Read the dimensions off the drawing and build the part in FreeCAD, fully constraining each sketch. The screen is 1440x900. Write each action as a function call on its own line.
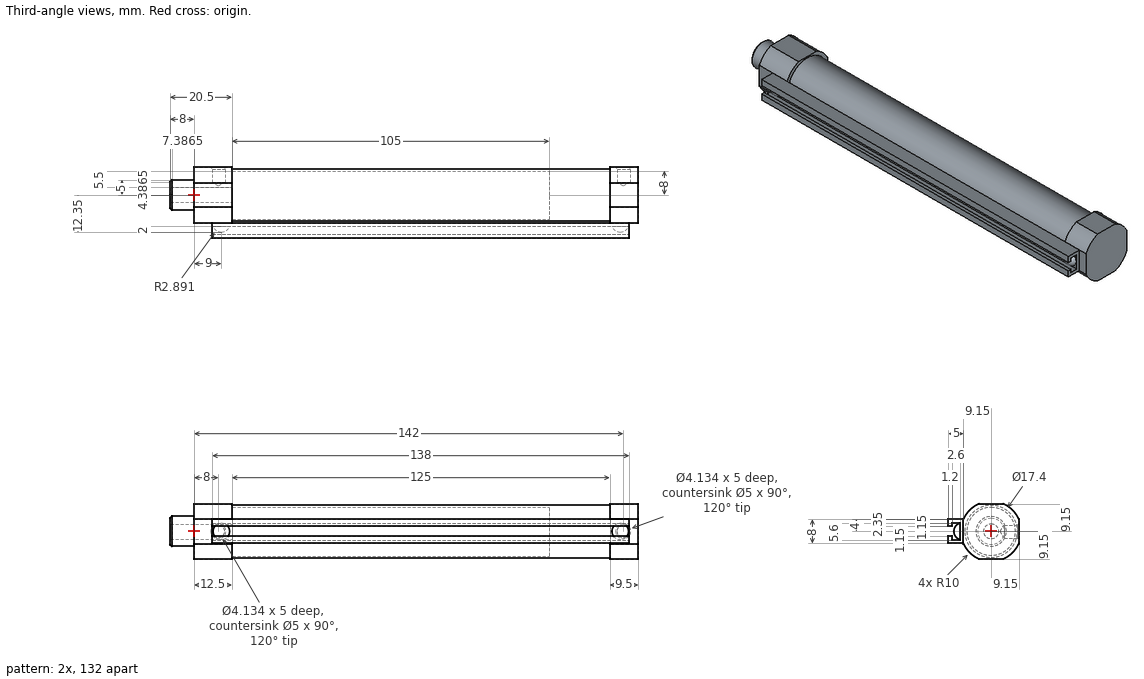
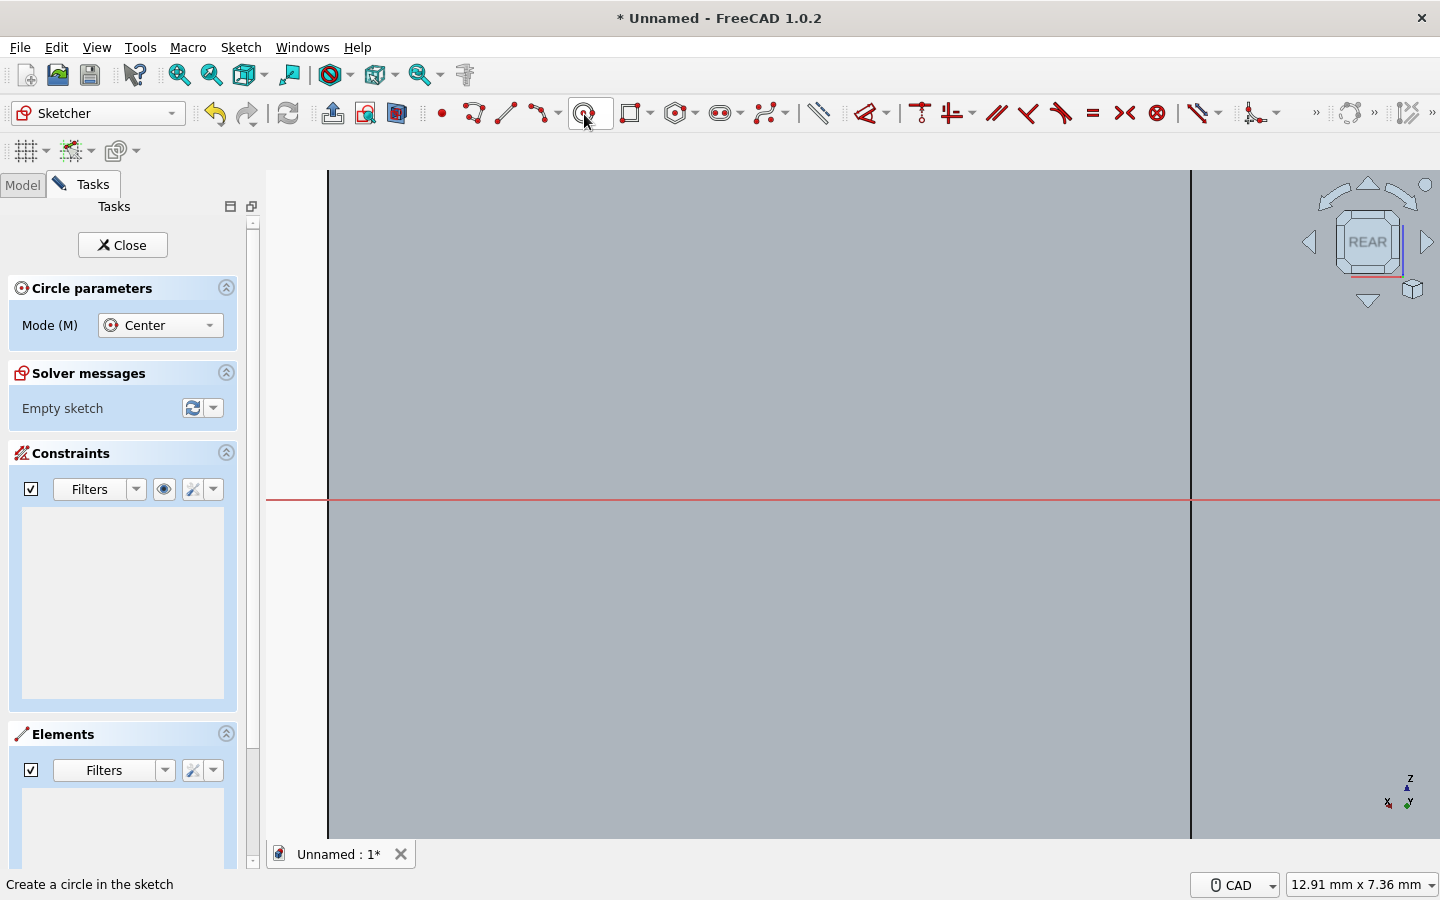
click(782, 500)
click(915, 367)
key(Escape)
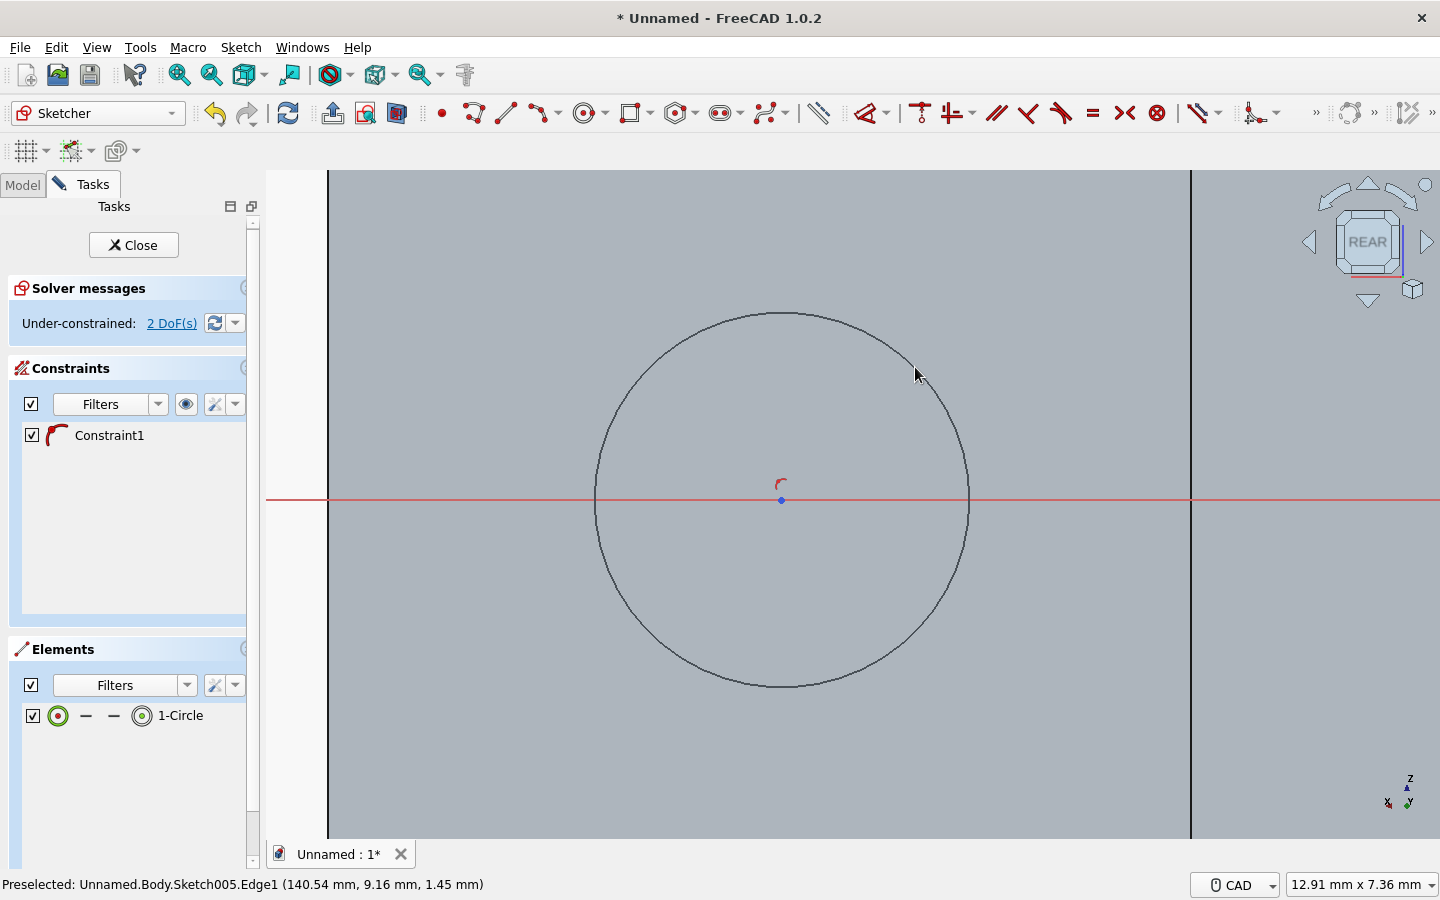
click(866, 114)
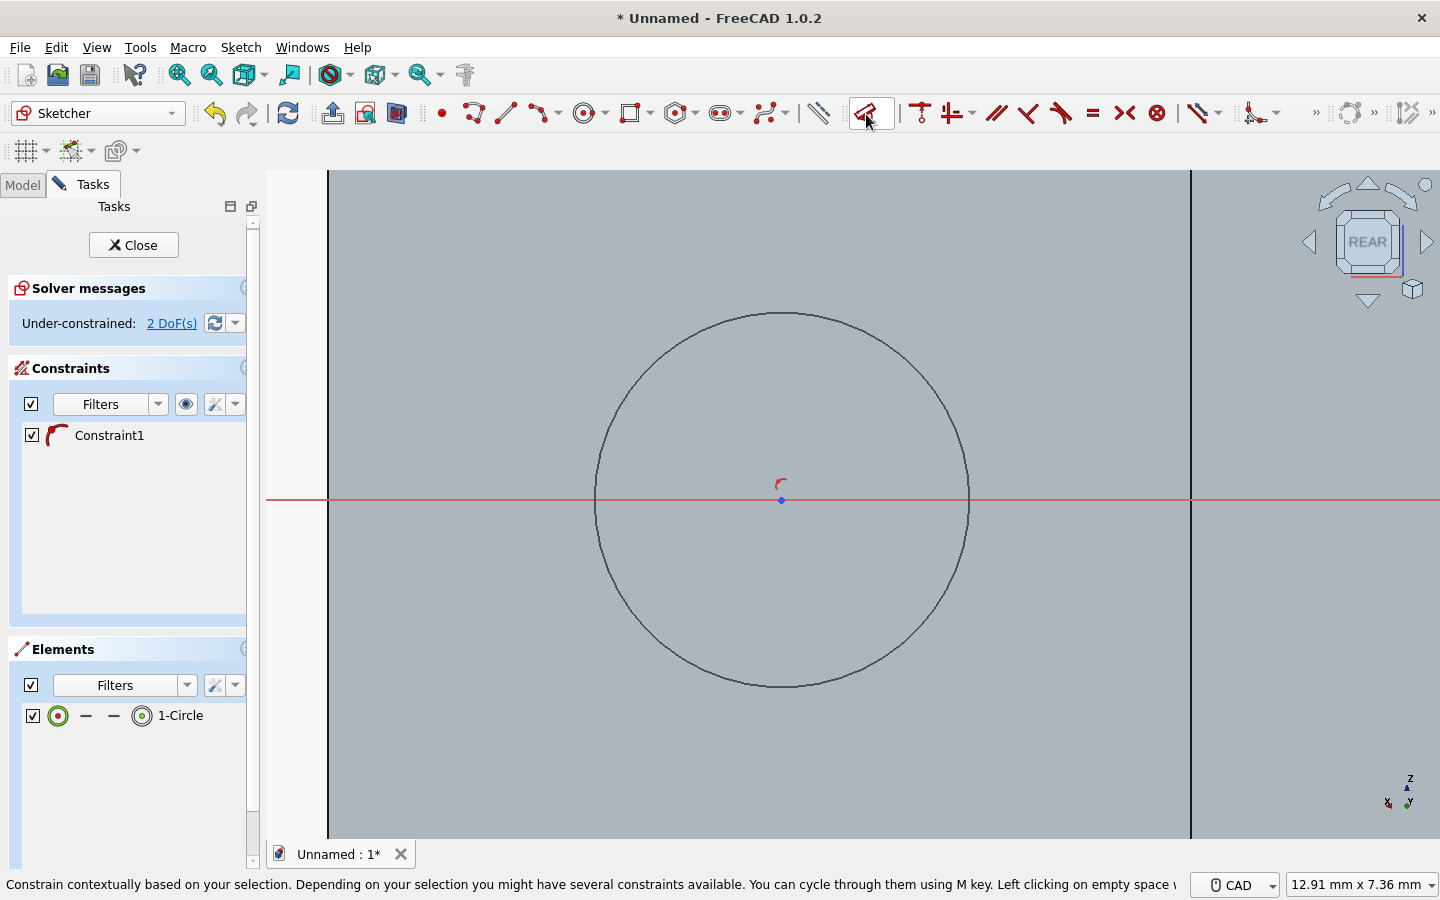
click(914, 367)
click(937, 344)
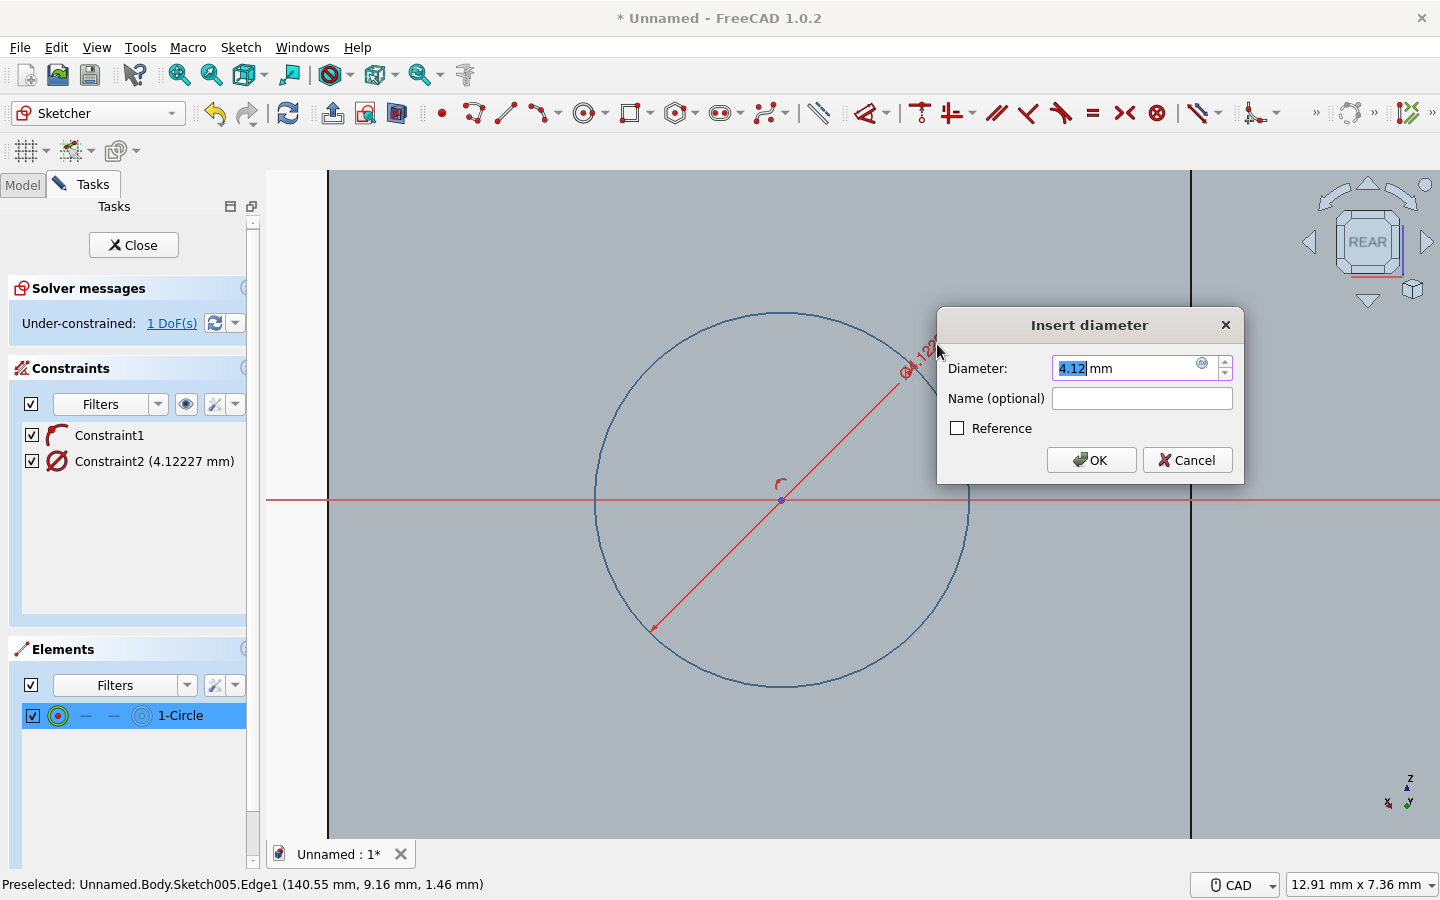
text(4.134)
key(Return)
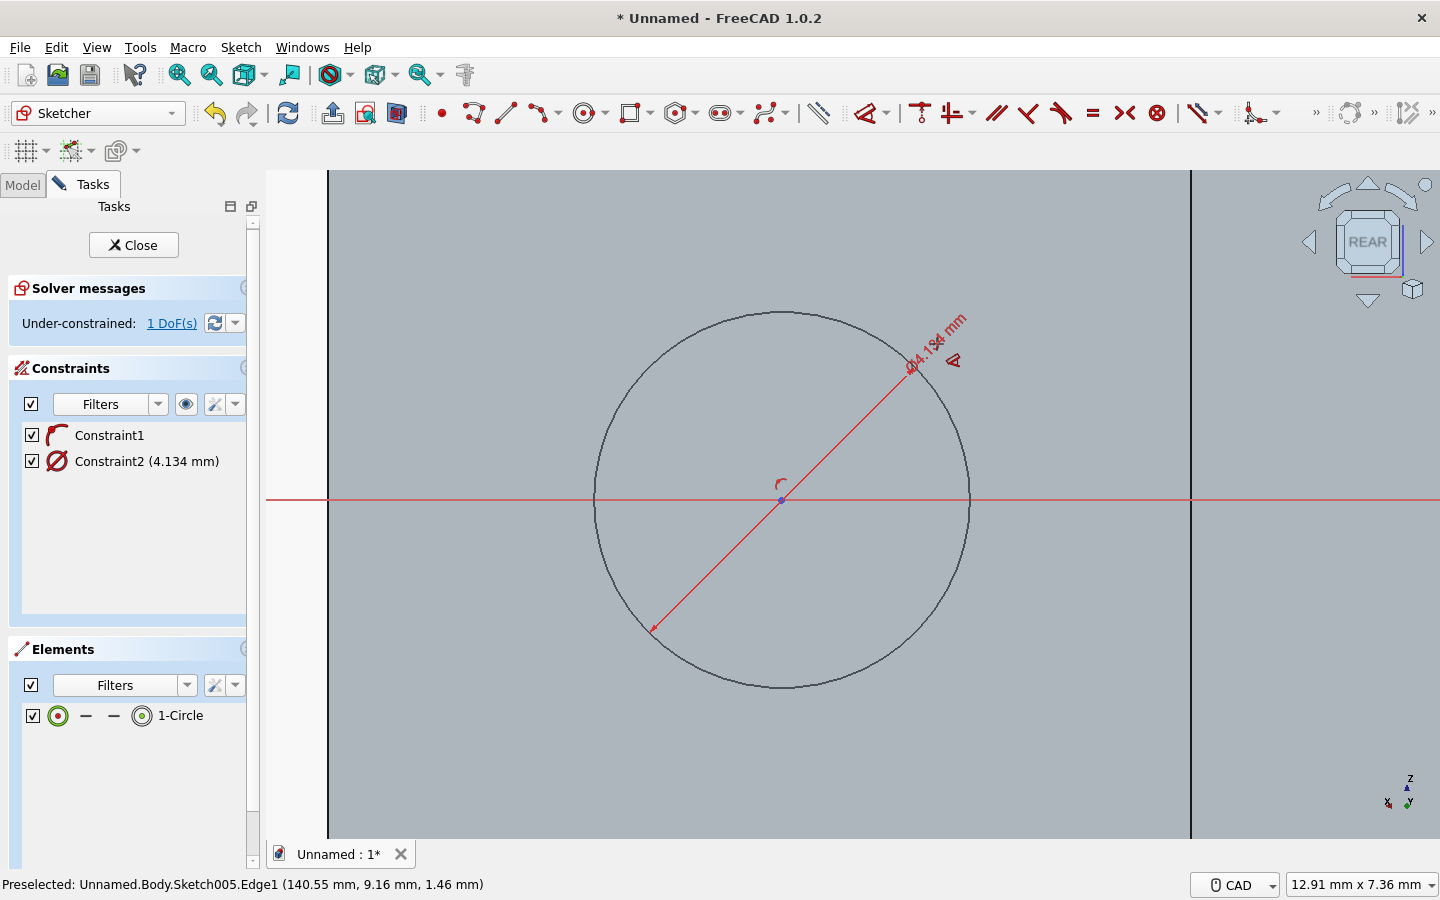
click(782, 500)
click(1028, 534)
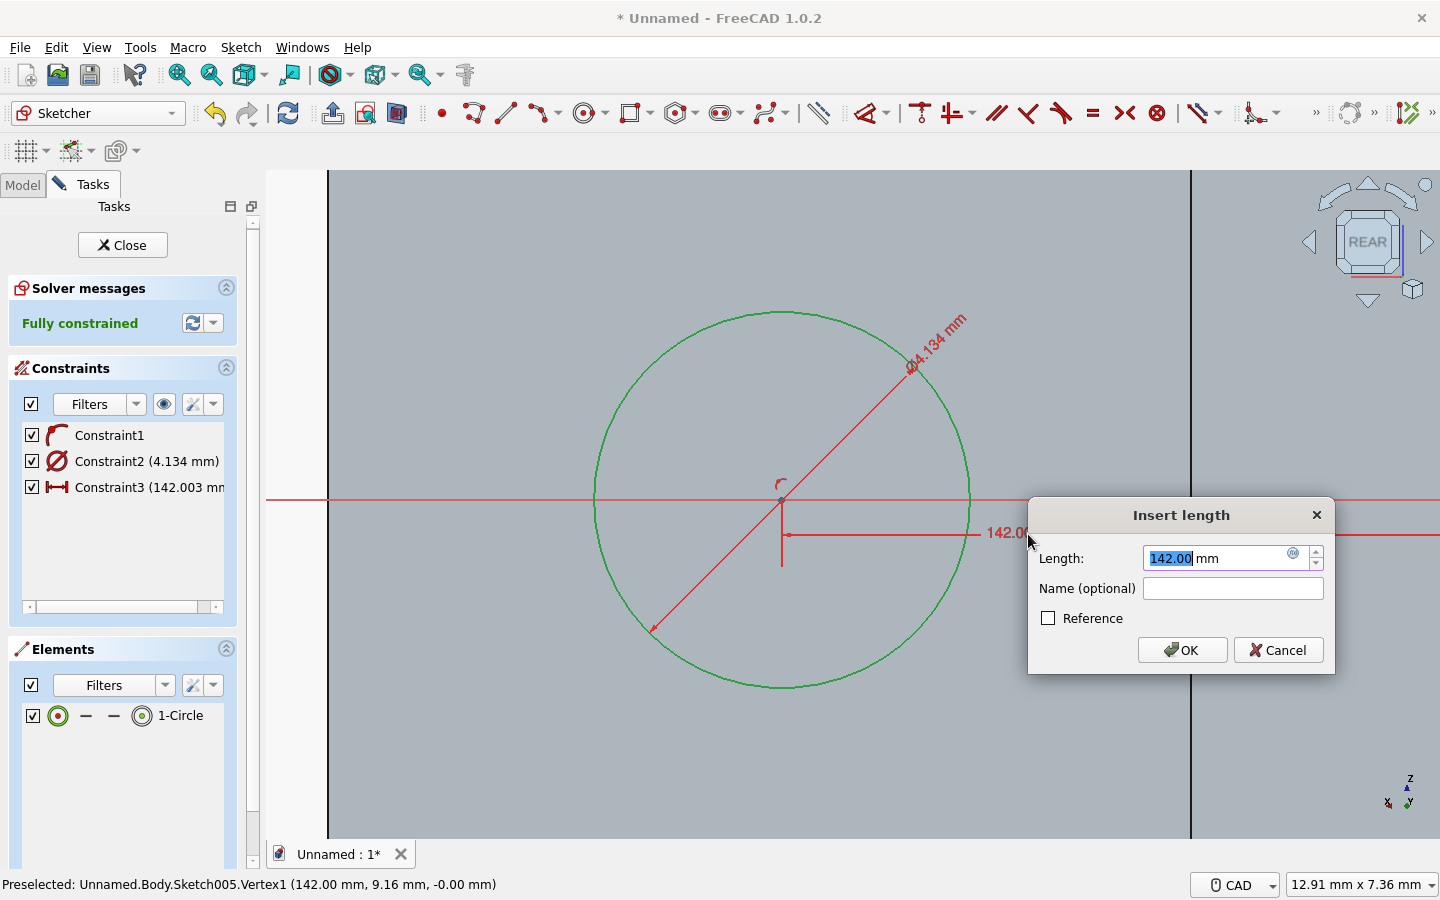
text(142)
key(Return)
key(Escape)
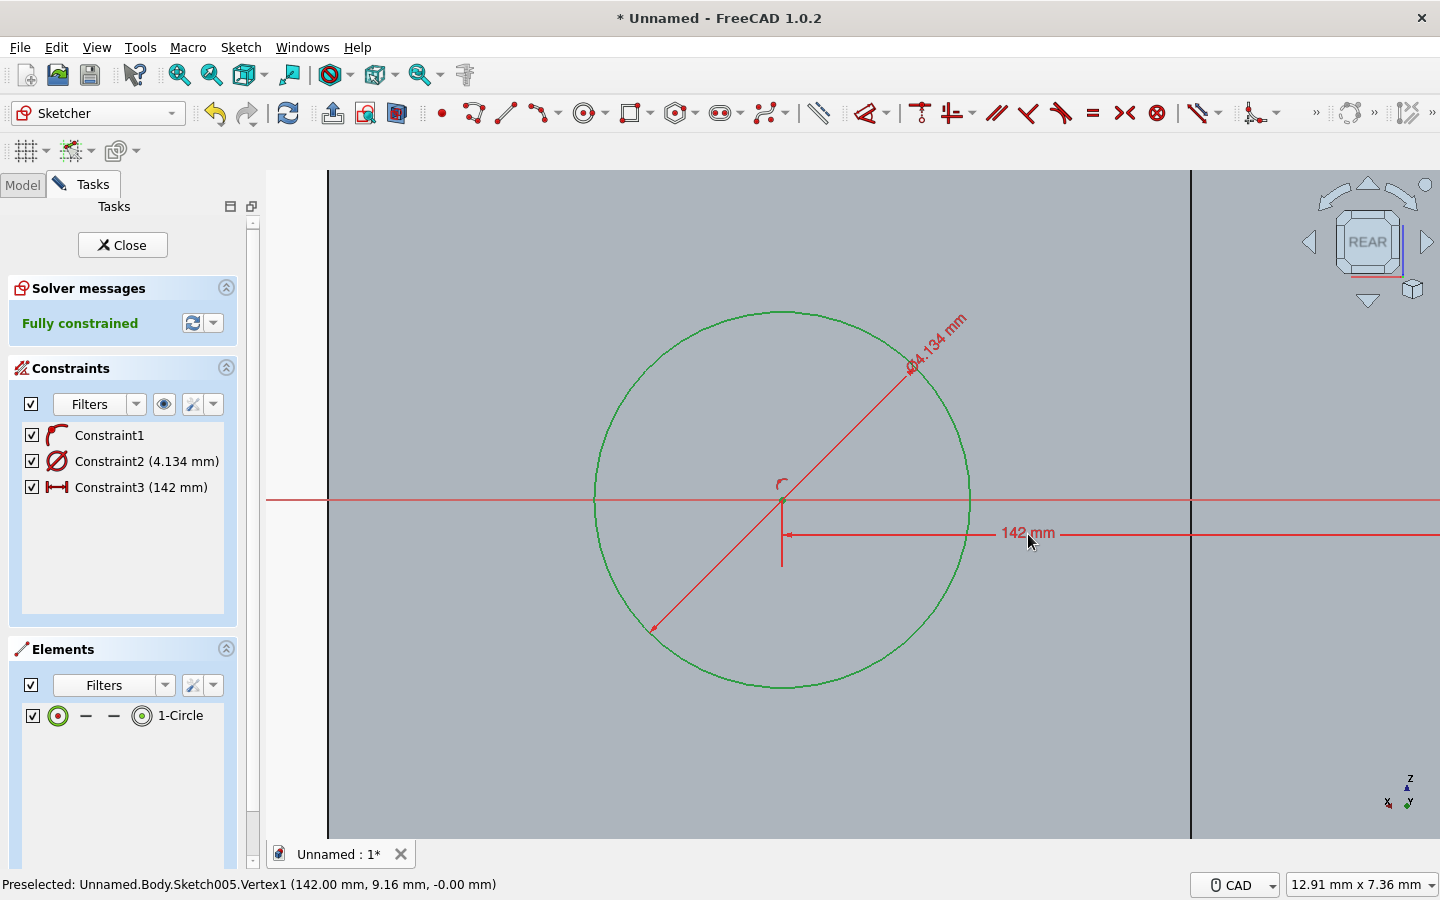
click(123, 245)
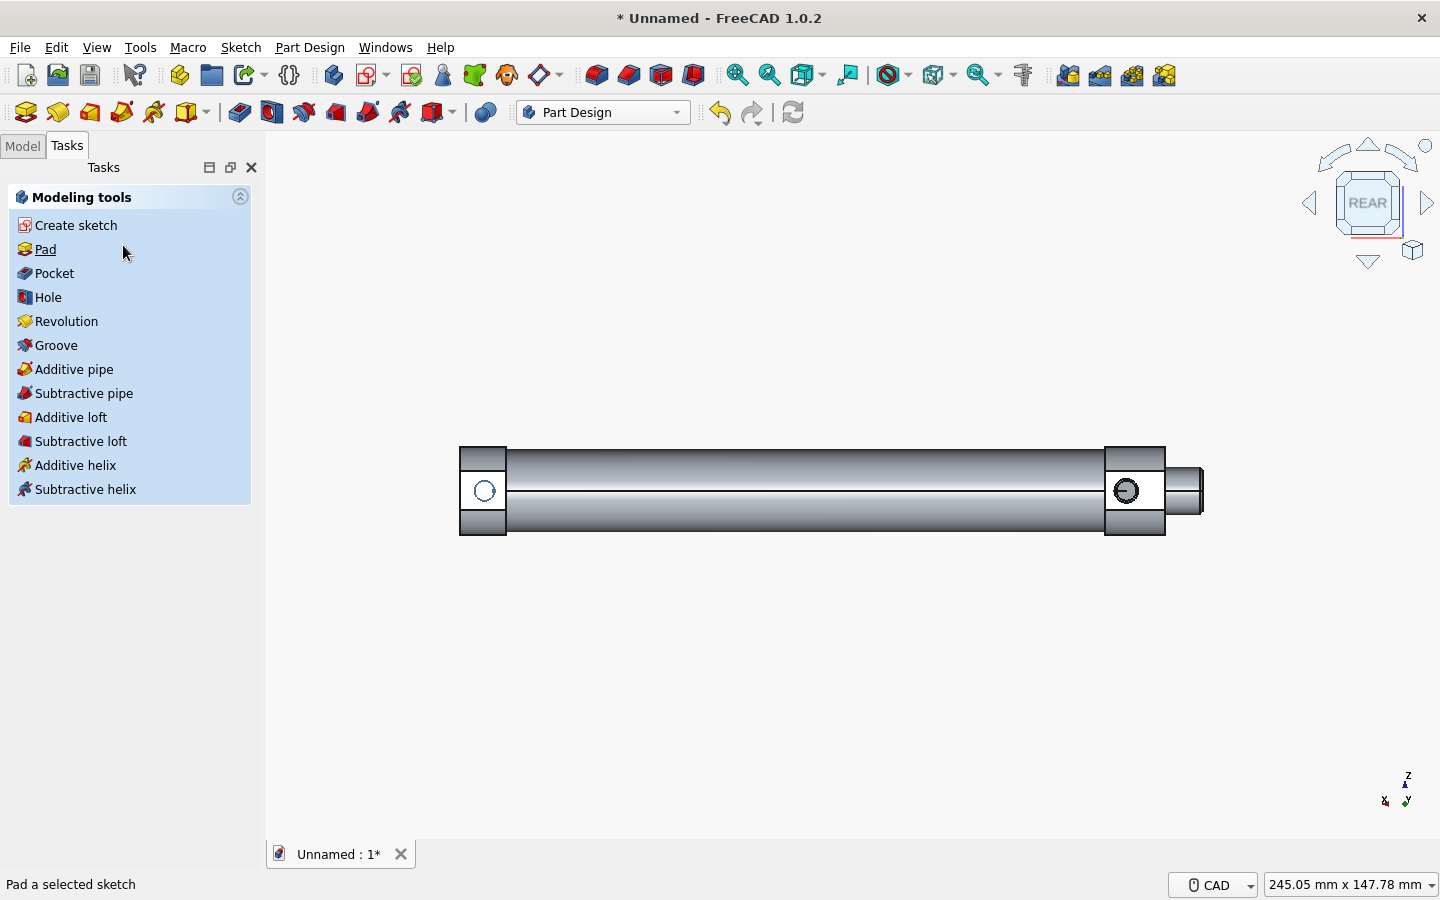
click(272, 112)